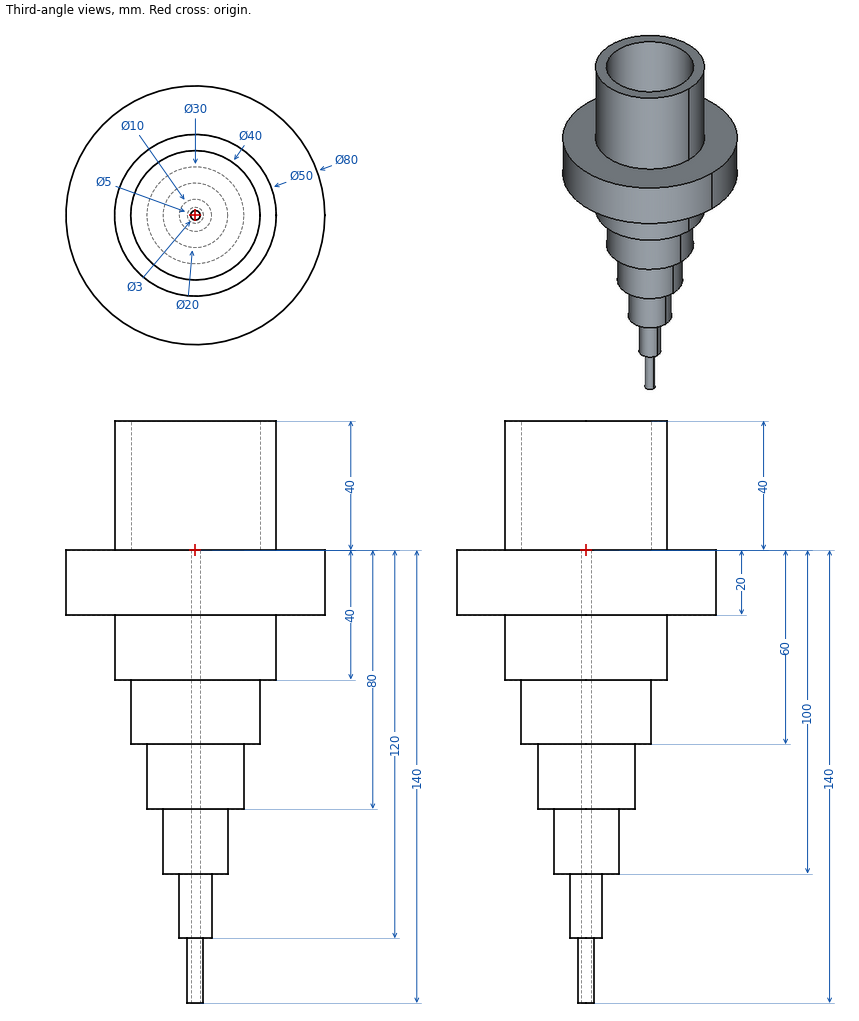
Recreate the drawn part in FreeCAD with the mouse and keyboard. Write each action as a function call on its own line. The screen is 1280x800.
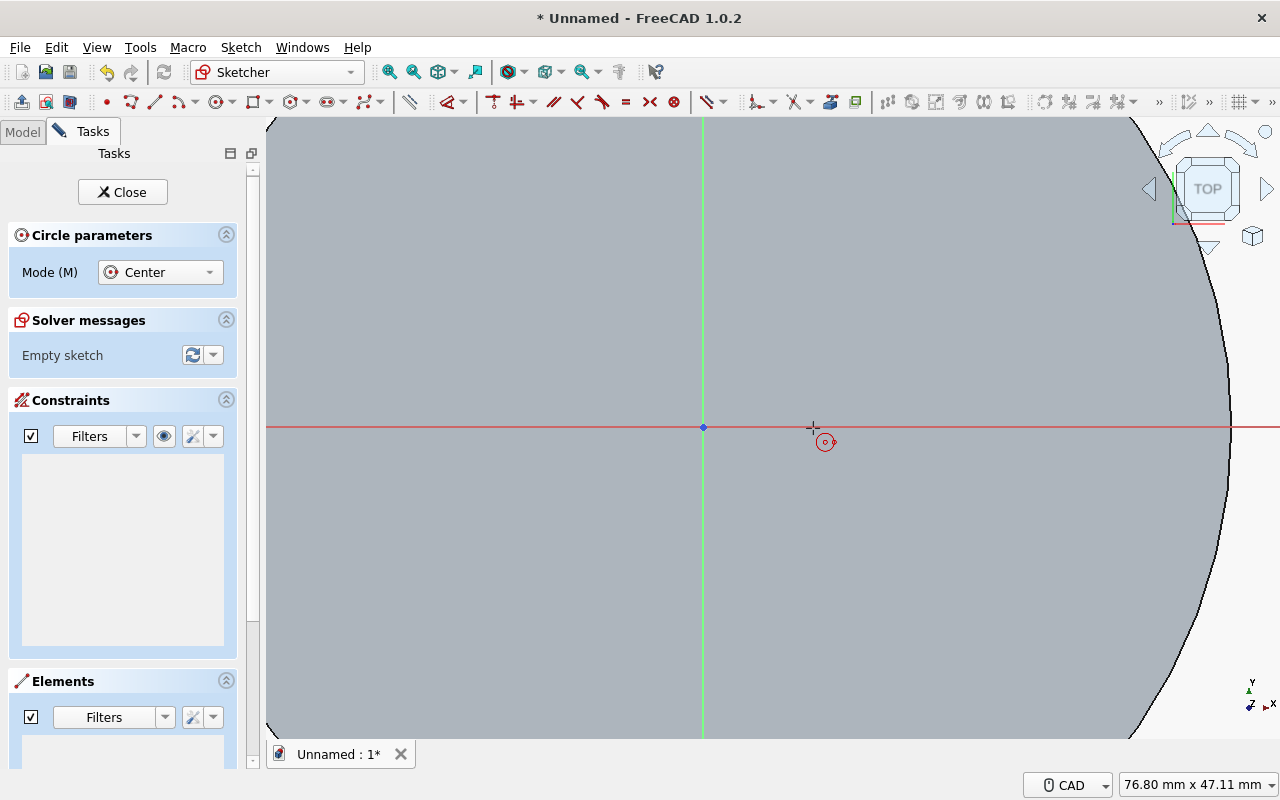
click(703, 427)
move(843, 287)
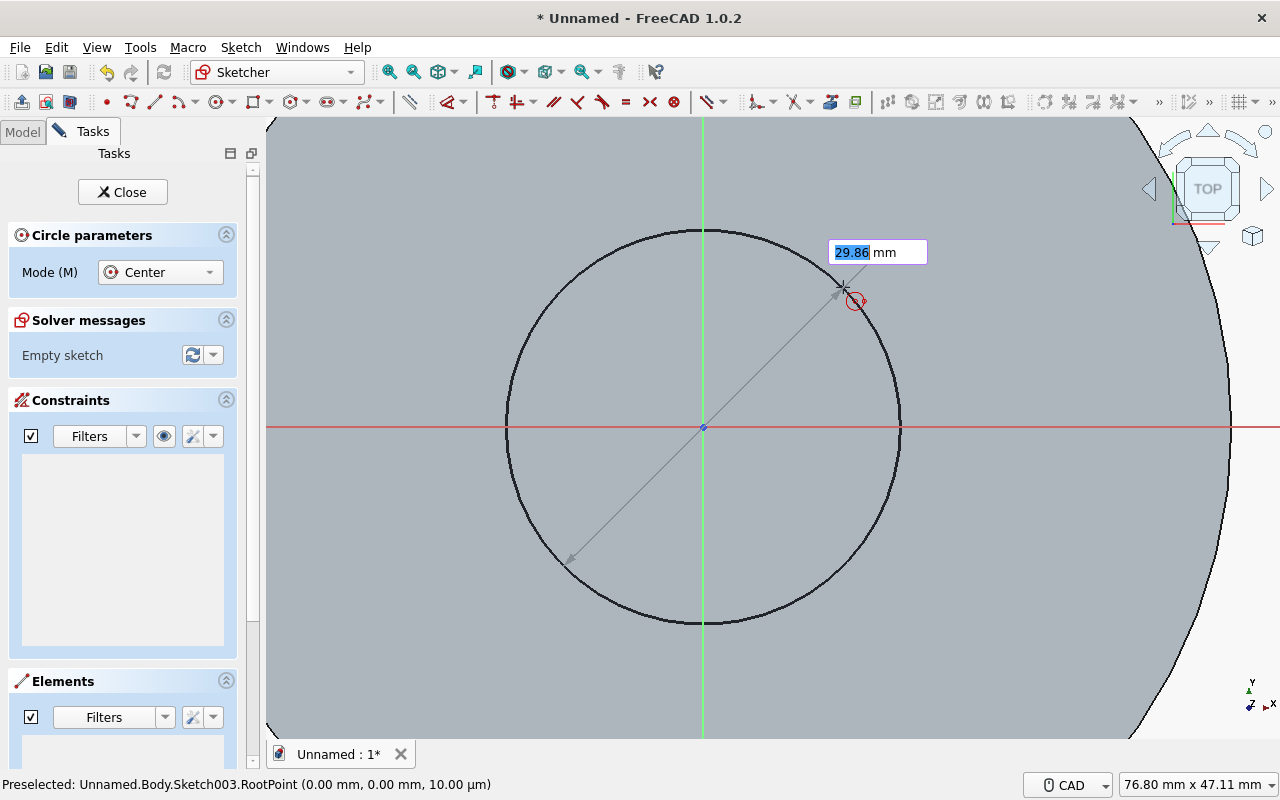
text(30)
key(Return)
key(Escape)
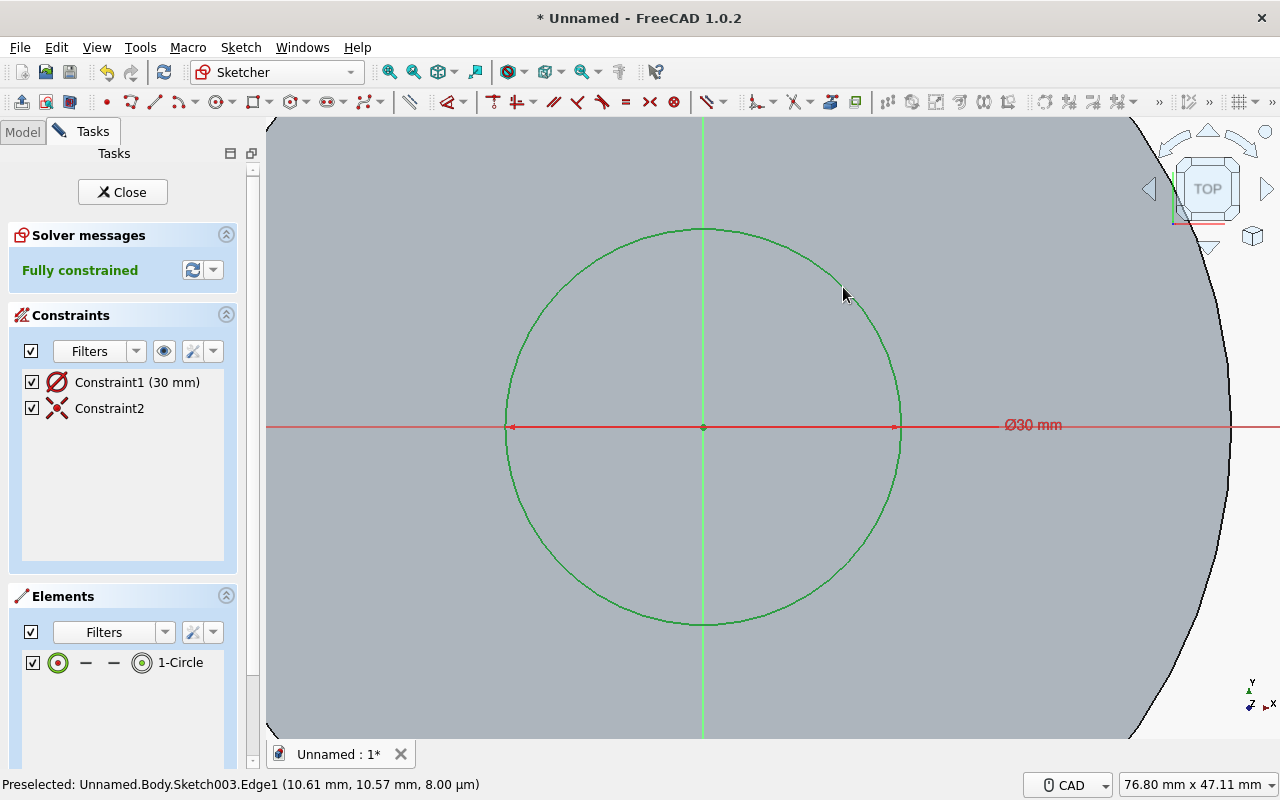
click(123, 192)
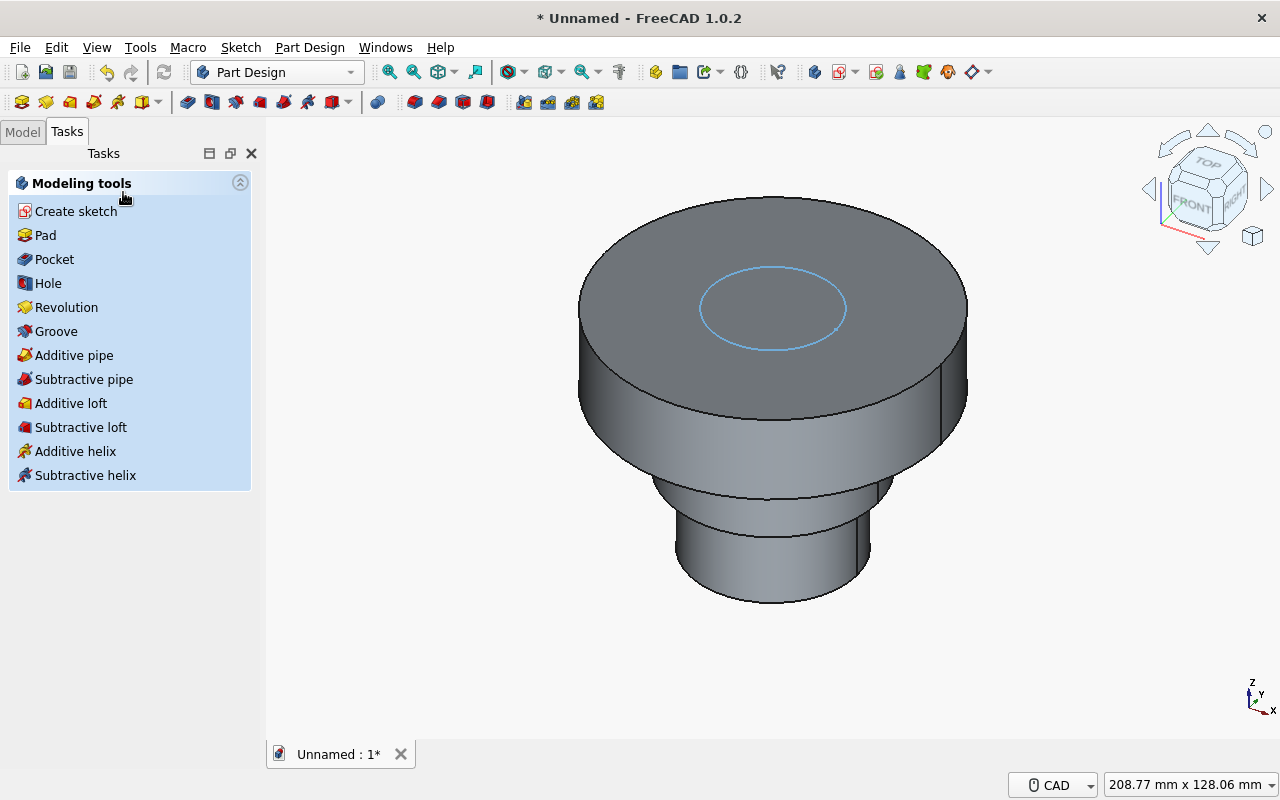
click(22, 102)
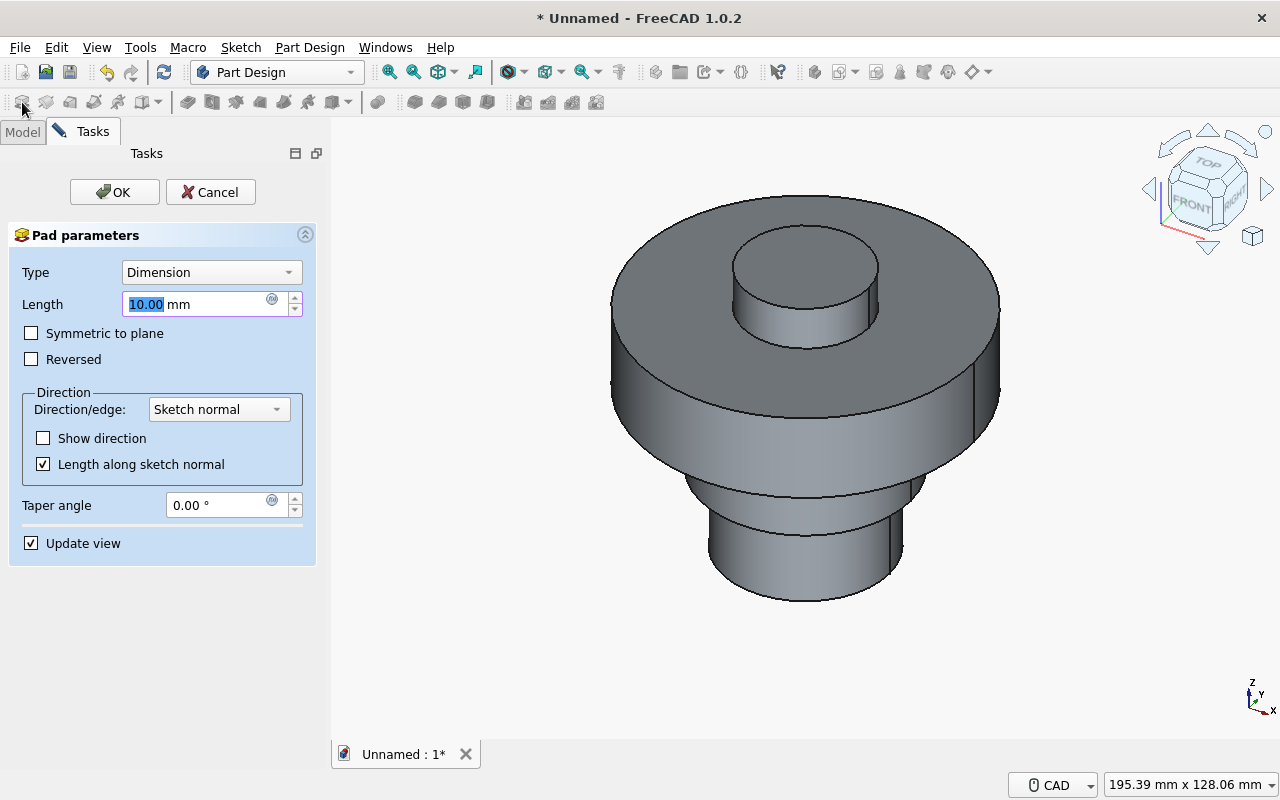
text(80)
key(Tab)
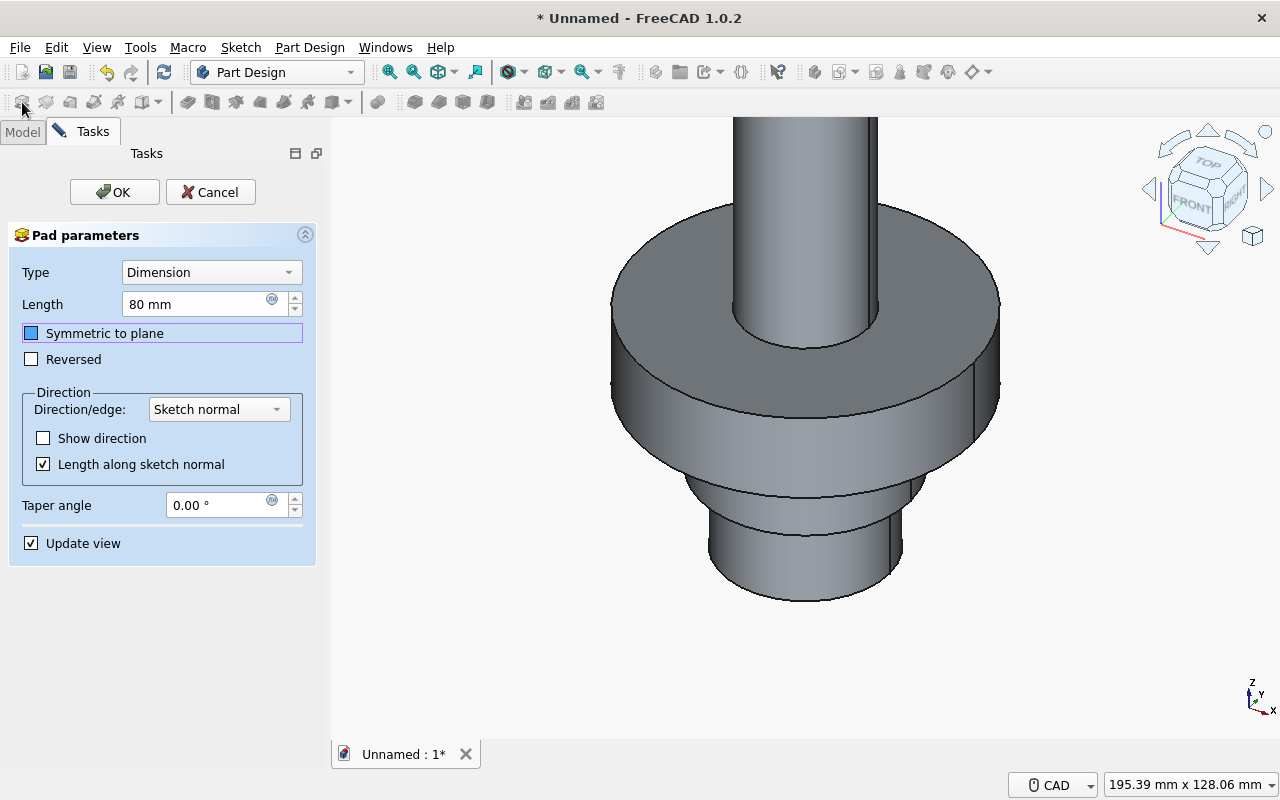
click(30, 359)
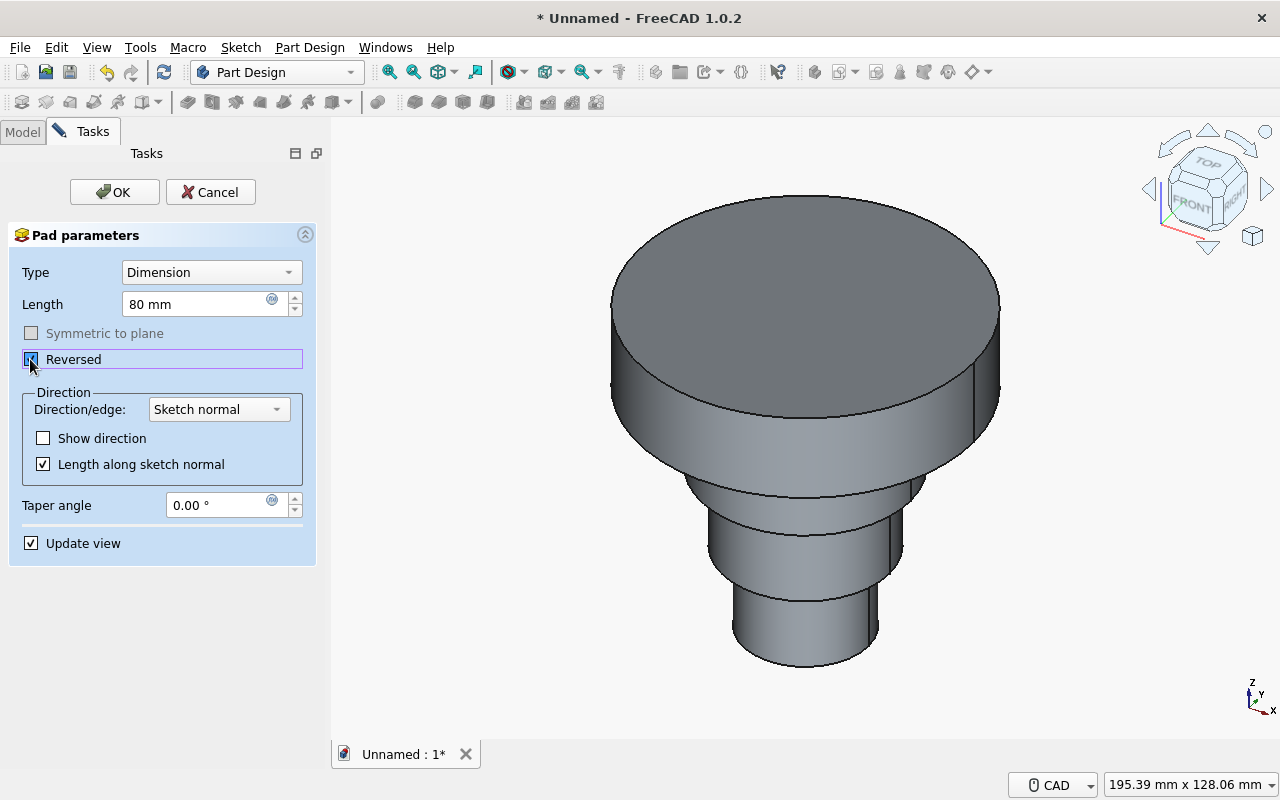
click(115, 192)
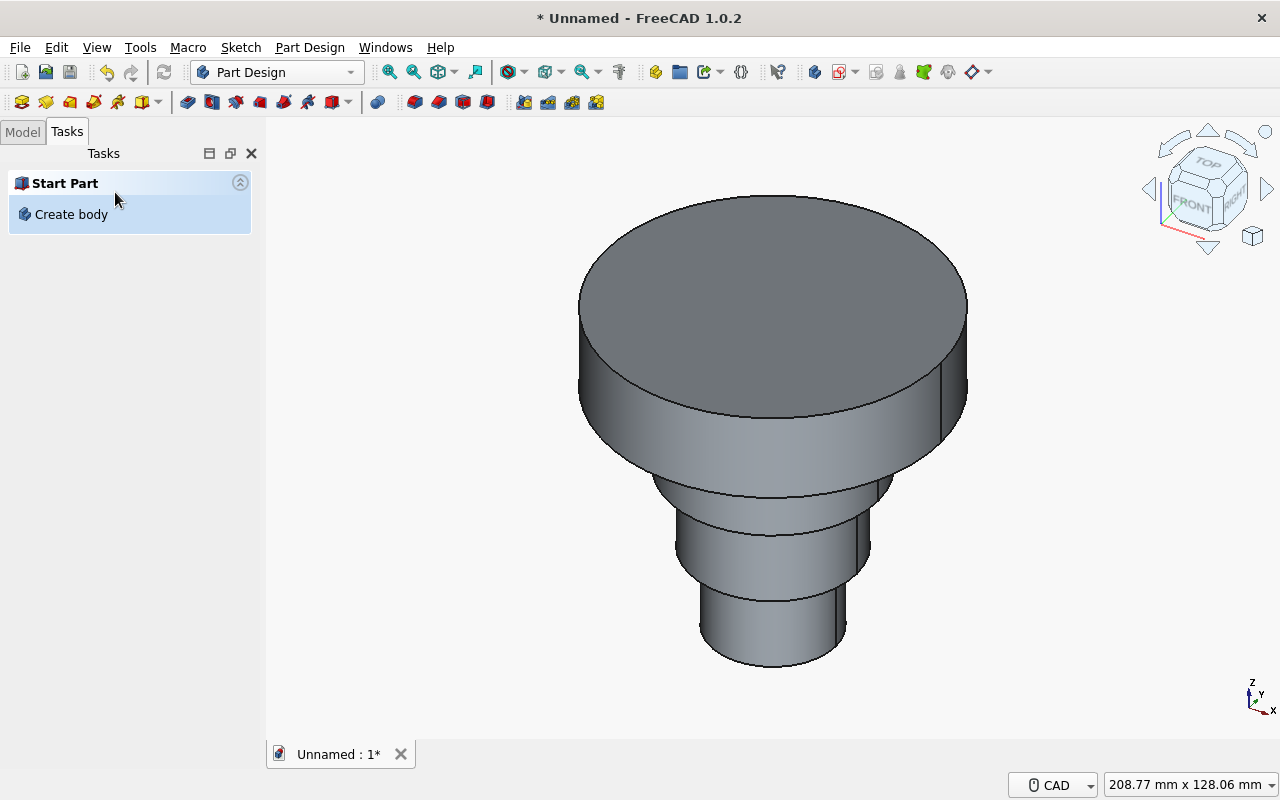
click(390, 72)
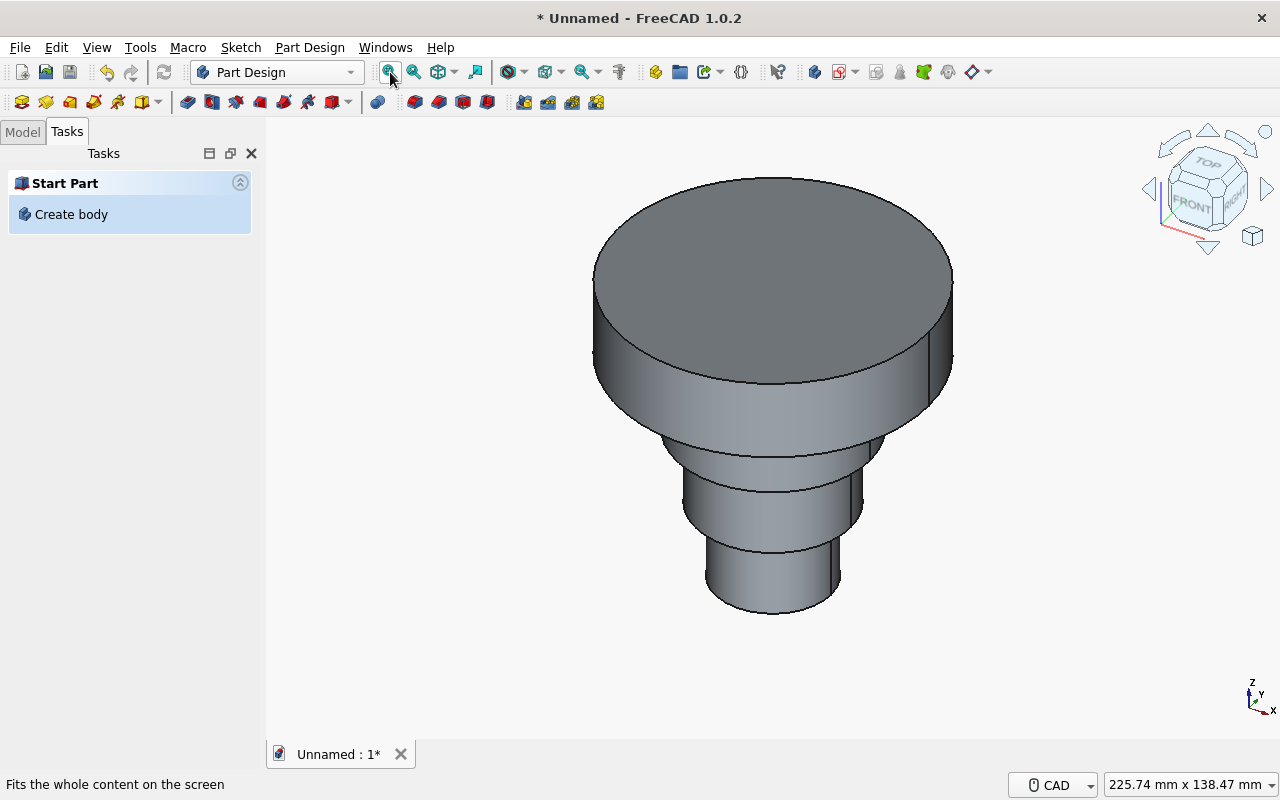
click(840, 72)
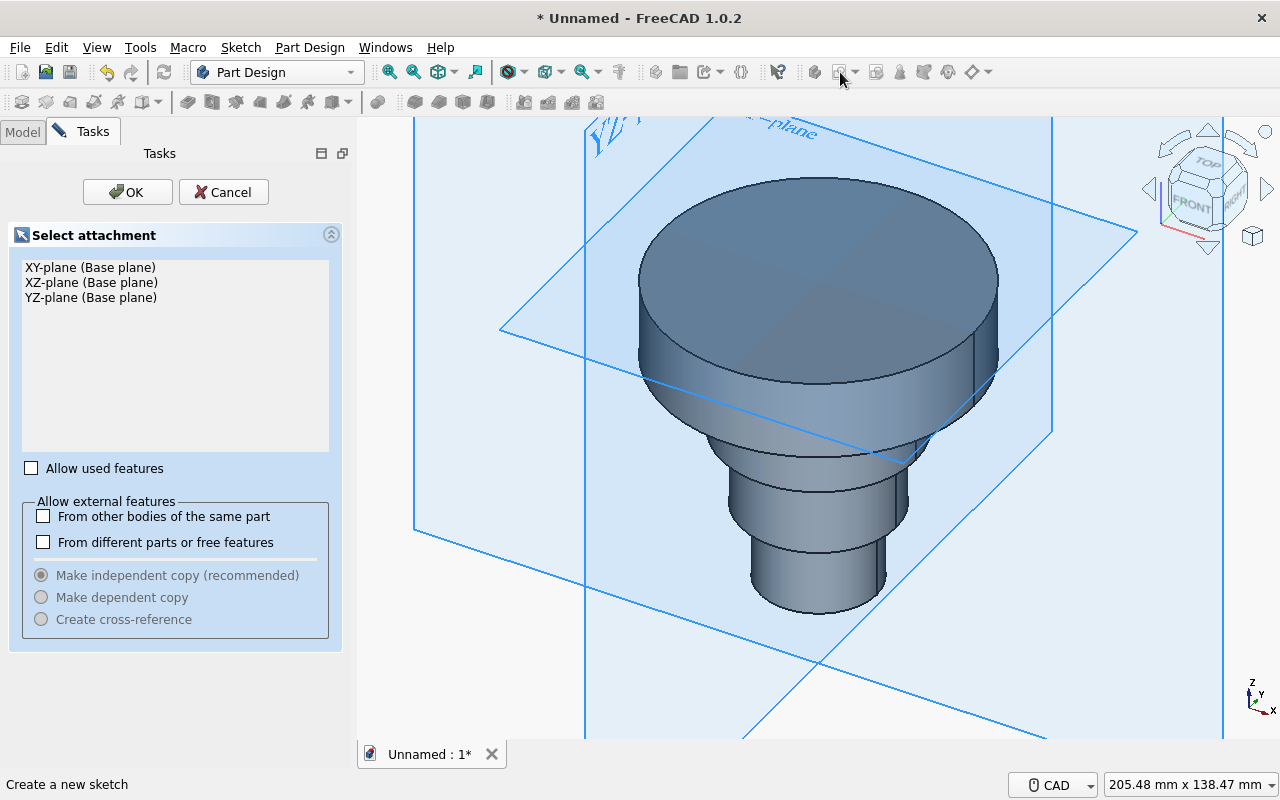
click(82, 268)